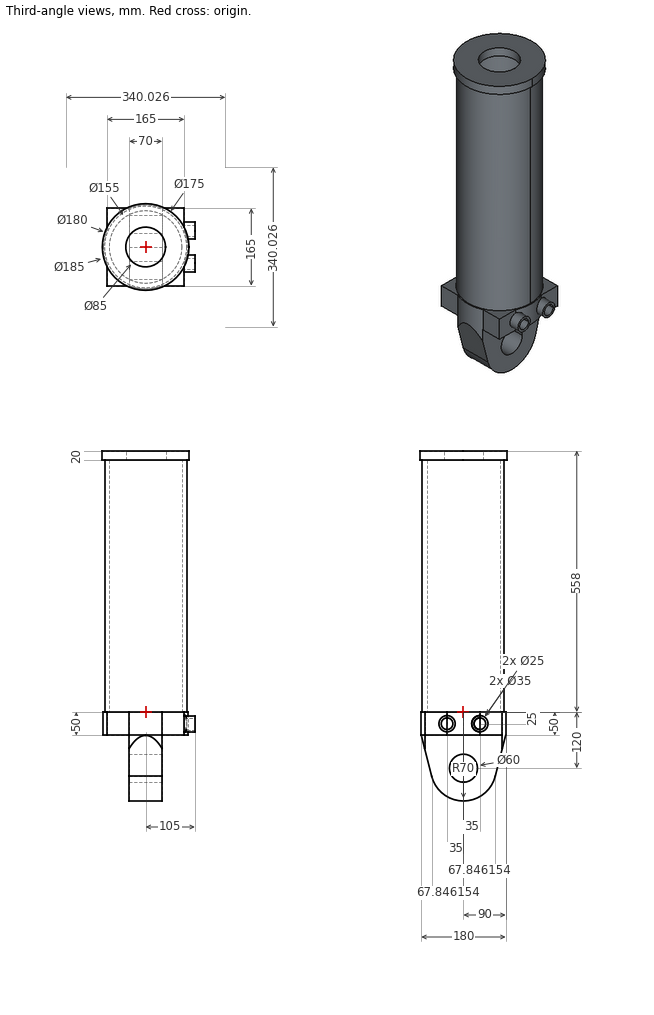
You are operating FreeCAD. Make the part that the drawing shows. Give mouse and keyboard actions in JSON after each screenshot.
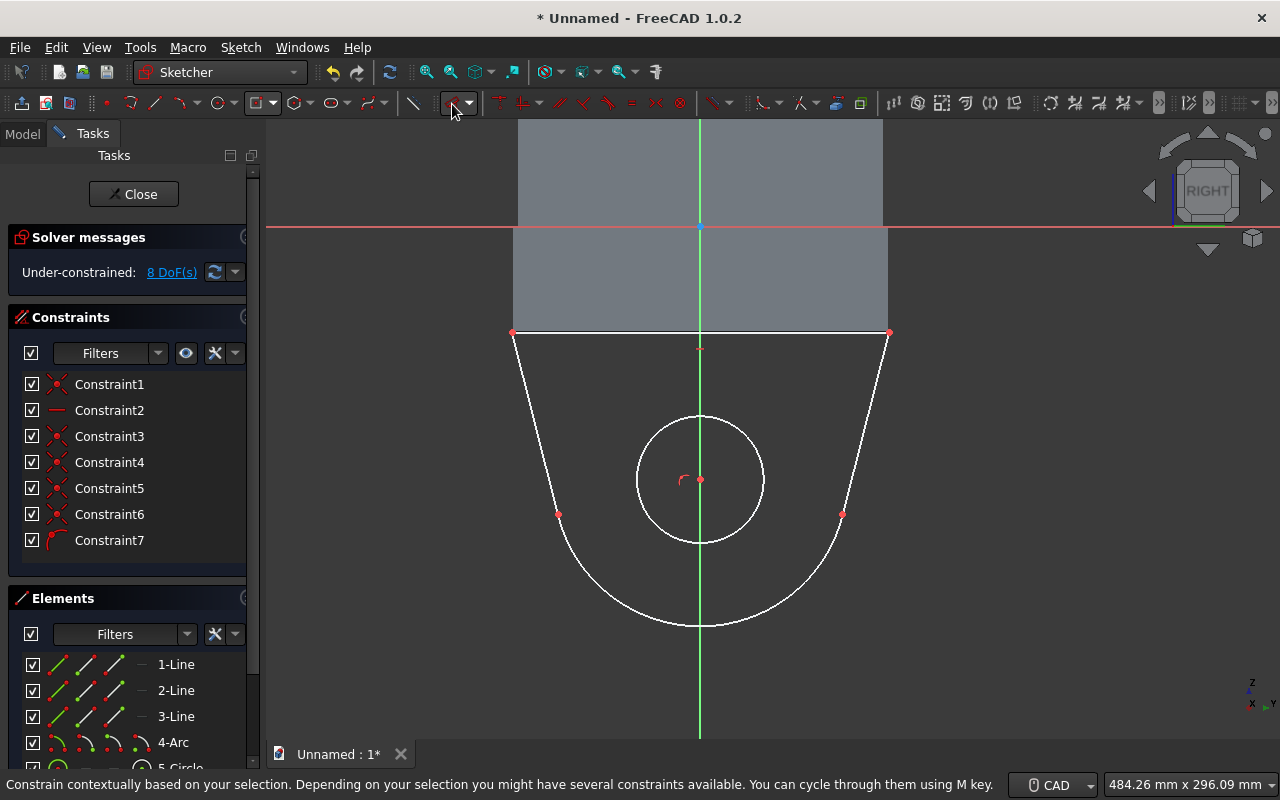
{"action": "left_click", "coordinate": [626, 606]}
{"action": "left_click", "coordinate": [610, 634]}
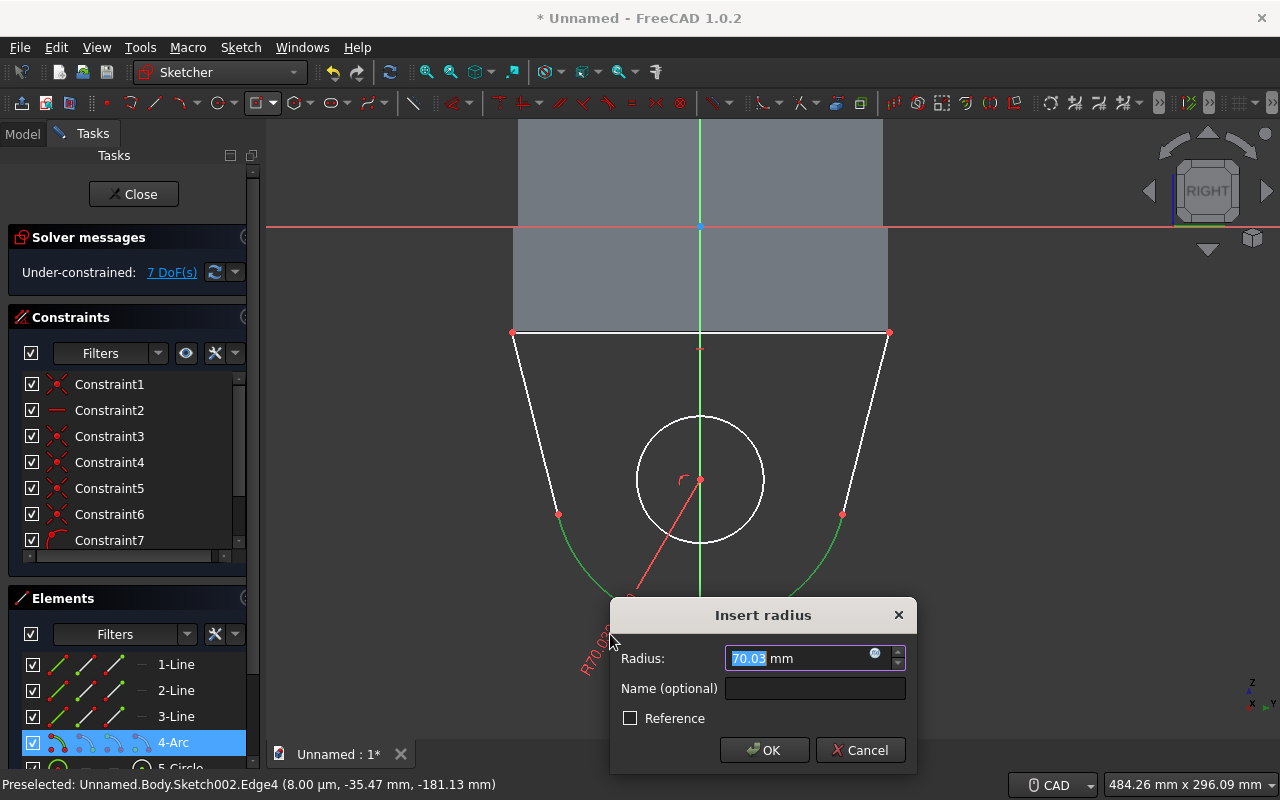
{"action": "type", "text": "70"}
{"action": "key", "text": "Return"}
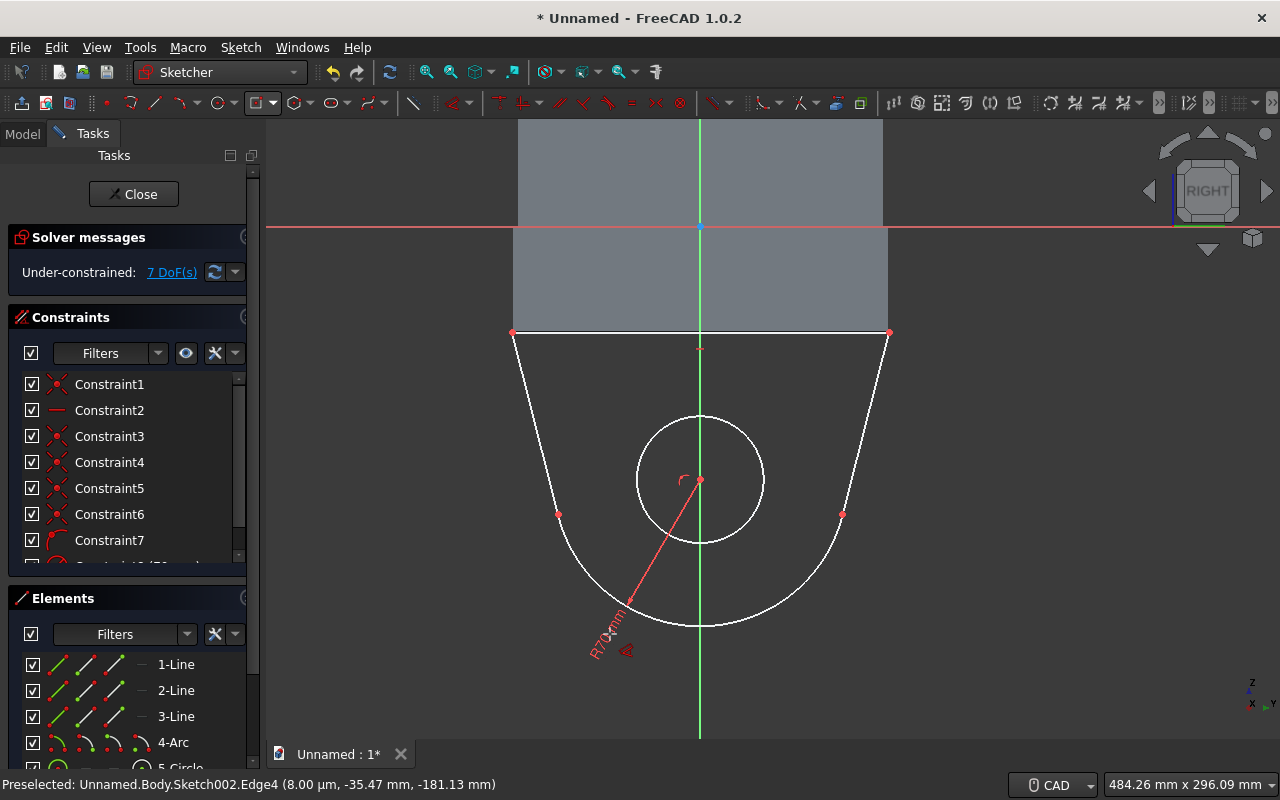
{"action": "left_click", "coordinate": [745, 435]}
{"action": "left_click", "coordinate": [768, 412]}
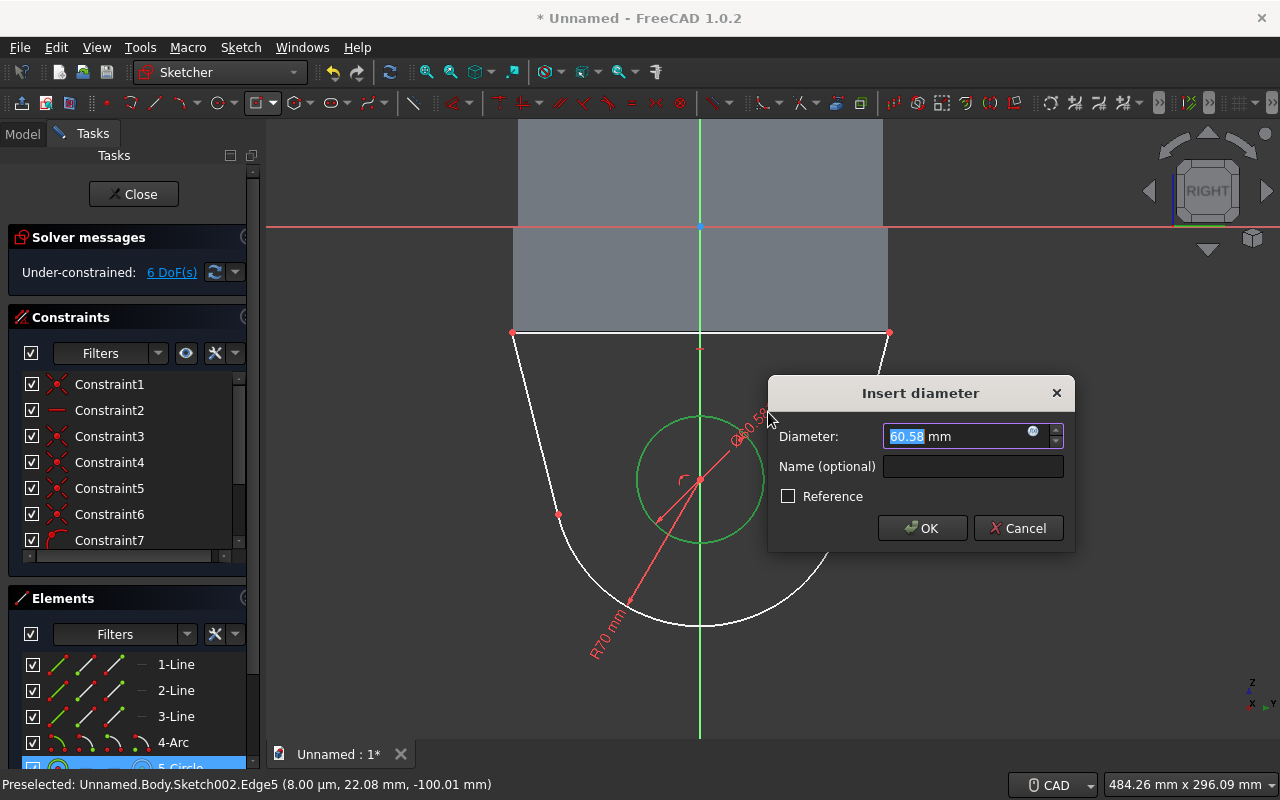
{"action": "type", "text": "60"}
{"action": "key", "text": "Return"}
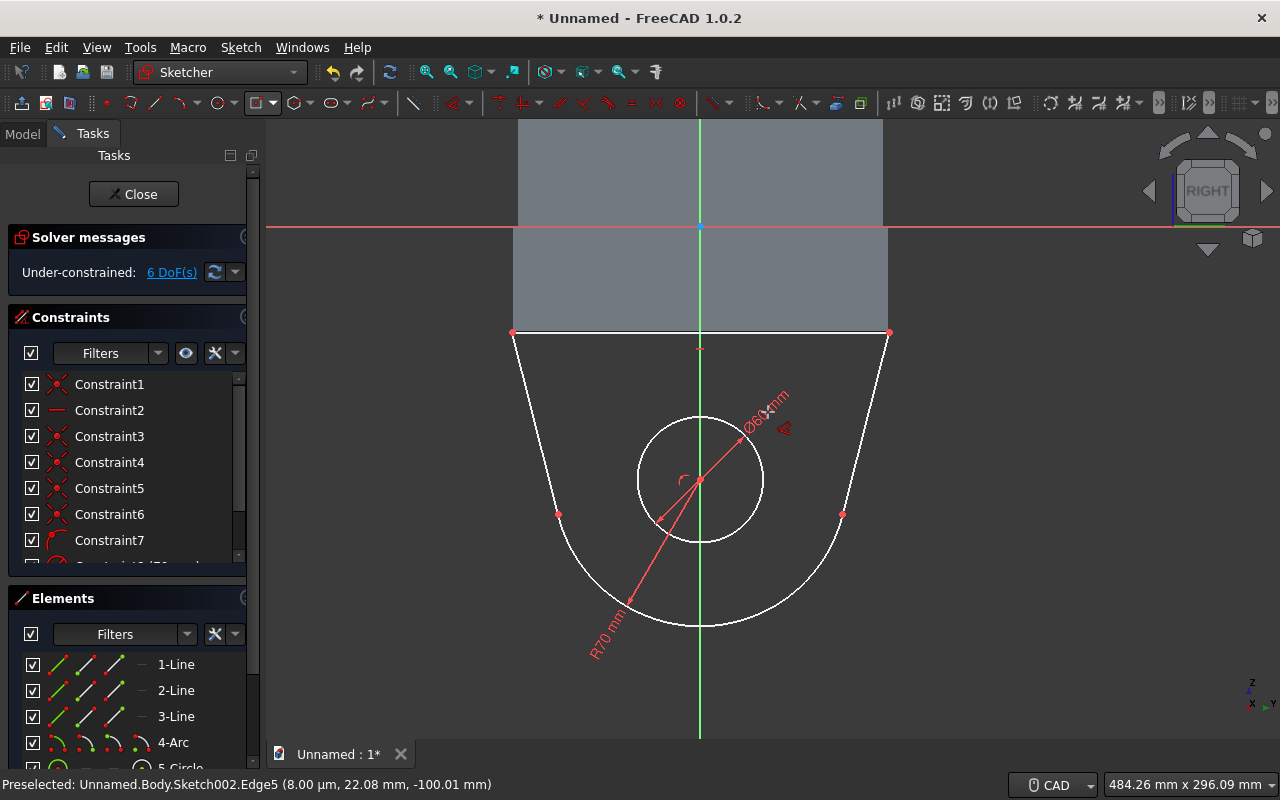
{"action": "left_click", "coordinate": [776, 333]}
{"action": "left_click", "coordinate": [614, 299]}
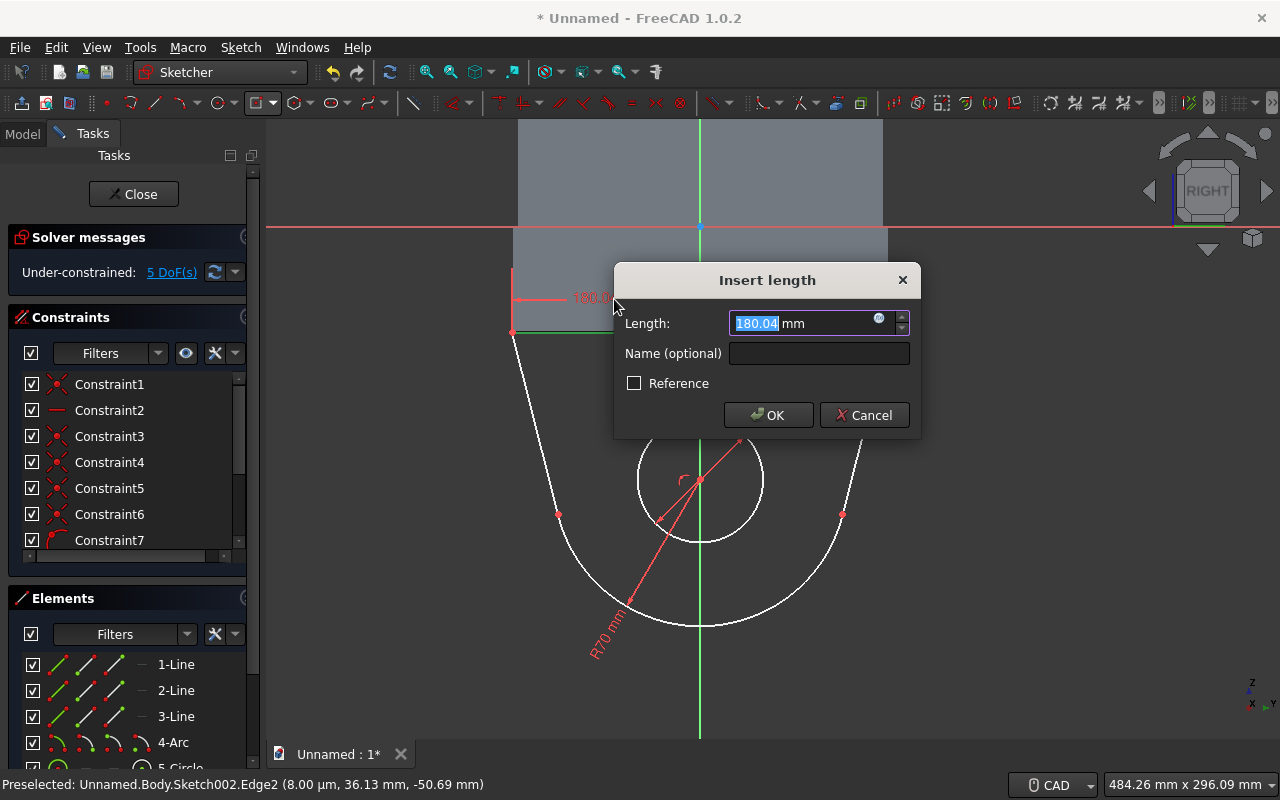
{"action": "type", "text": "180"}
{"action": "key", "text": "Return"}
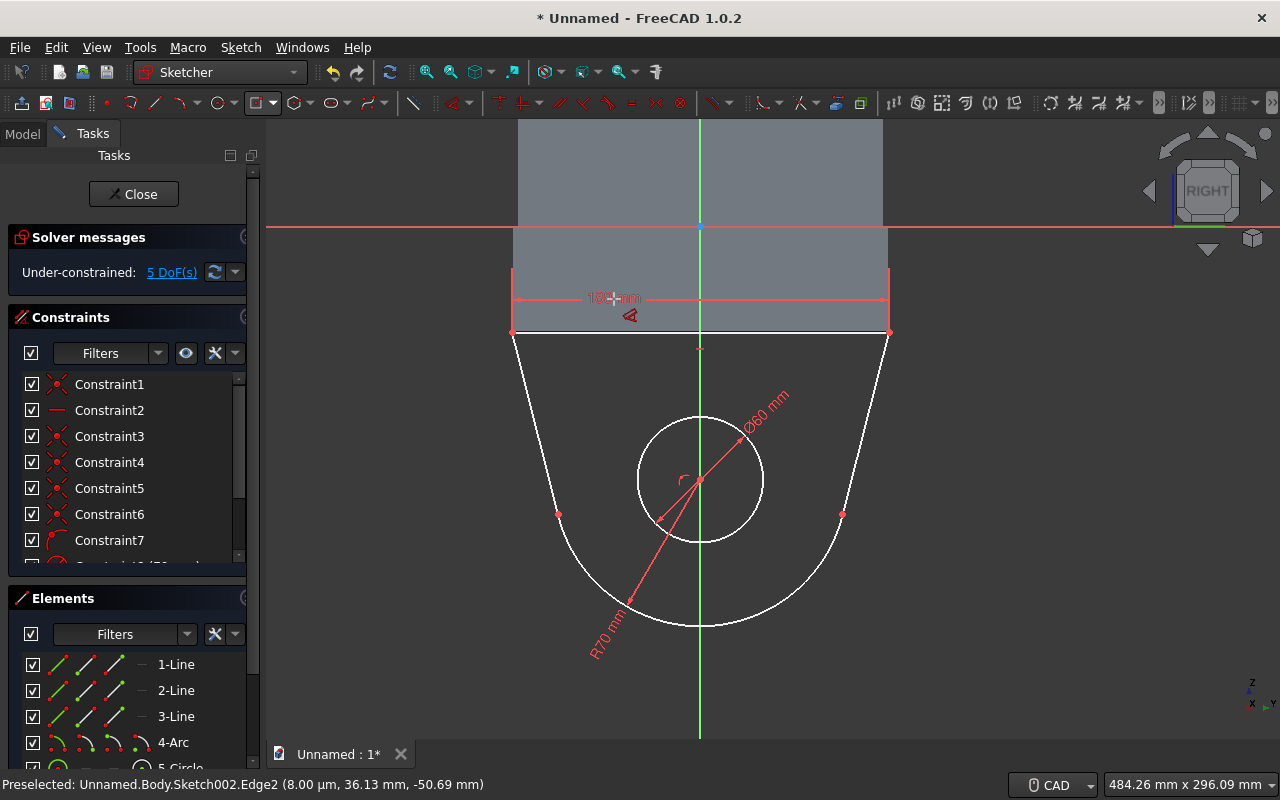
{"action": "left_click", "coordinate": [889, 333]}
{"action": "left_click", "coordinate": [795, 193]}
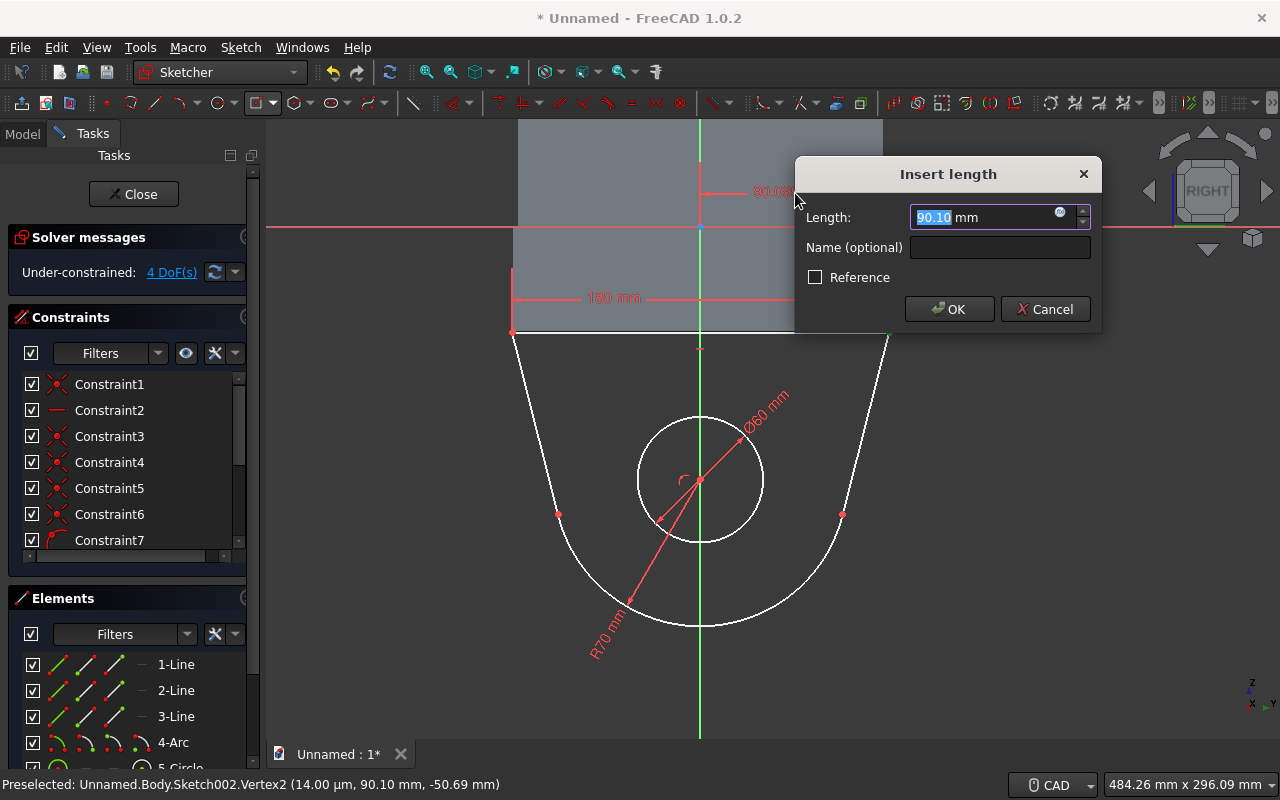
{"action": "type", "text": "90"}
{"action": "key", "text": "Return"}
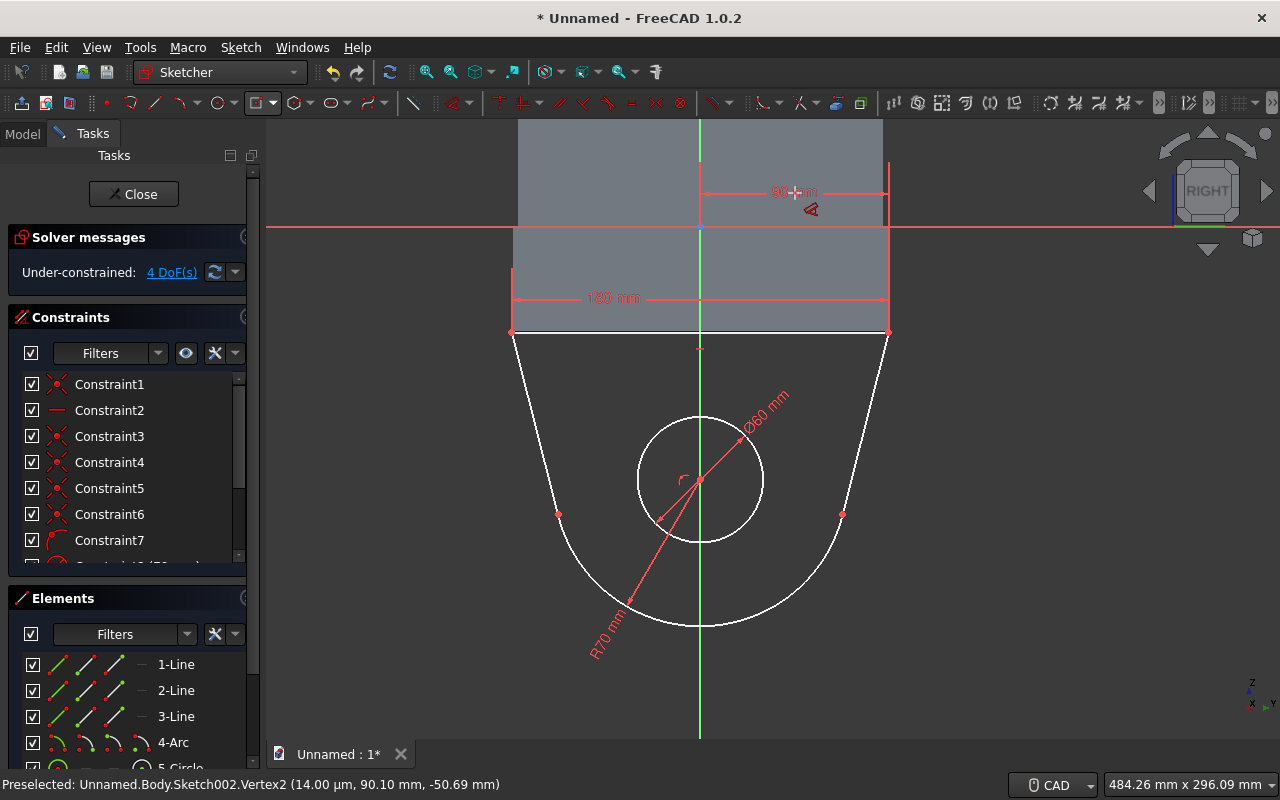
{"action": "left_click", "coordinate": [889, 333]}
{"action": "left_click", "coordinate": [923, 280]}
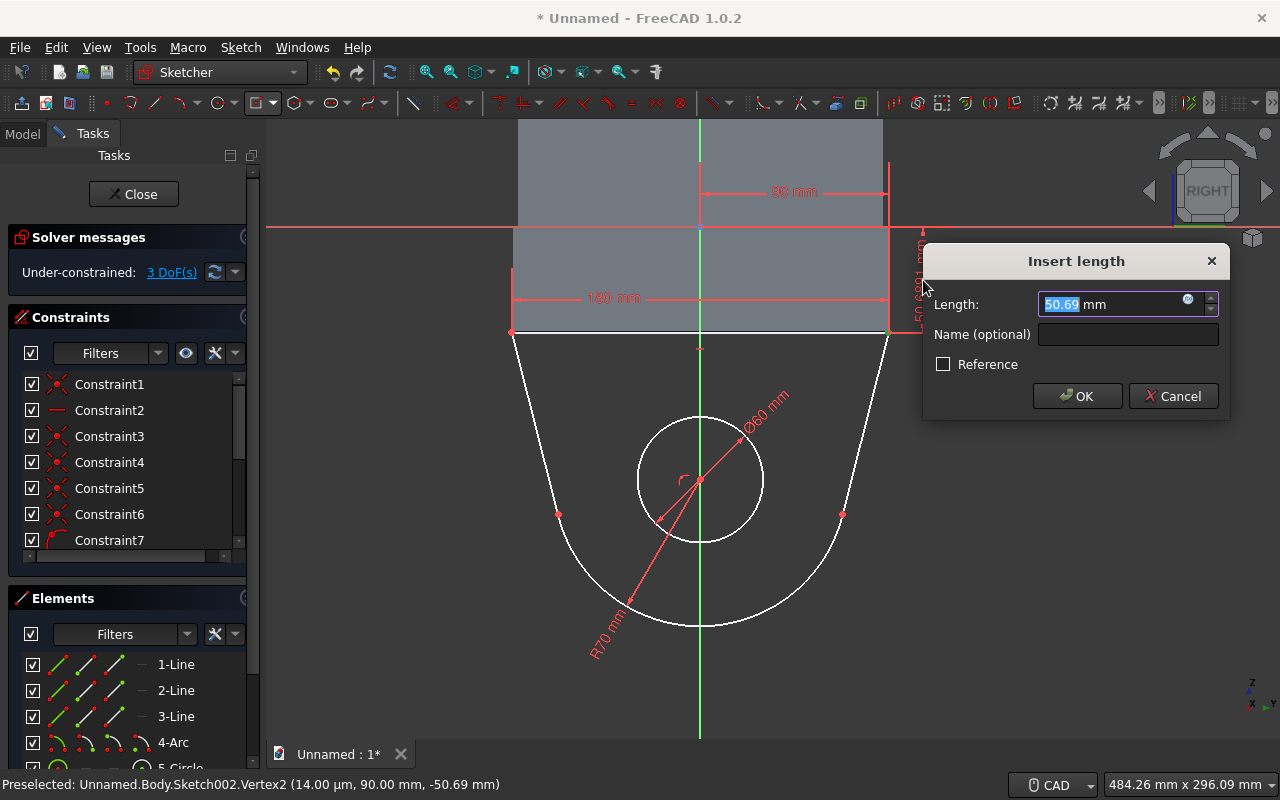
{"action": "type", "text": "50"}
{"action": "key", "text": "Return"}